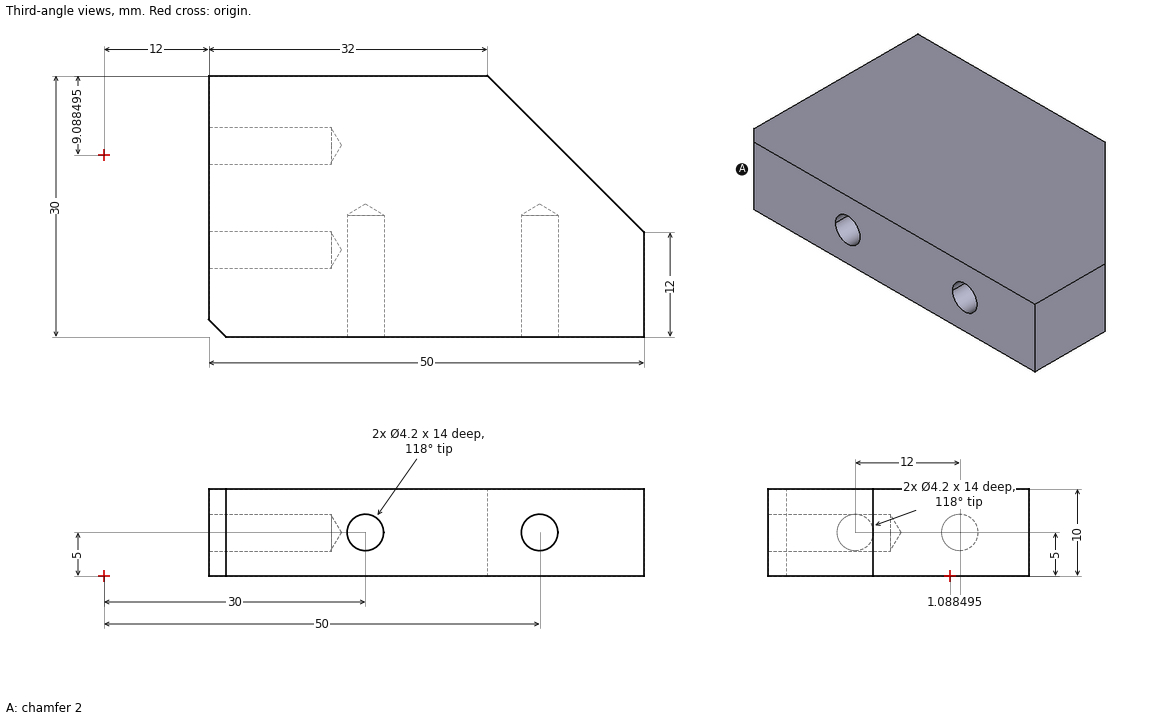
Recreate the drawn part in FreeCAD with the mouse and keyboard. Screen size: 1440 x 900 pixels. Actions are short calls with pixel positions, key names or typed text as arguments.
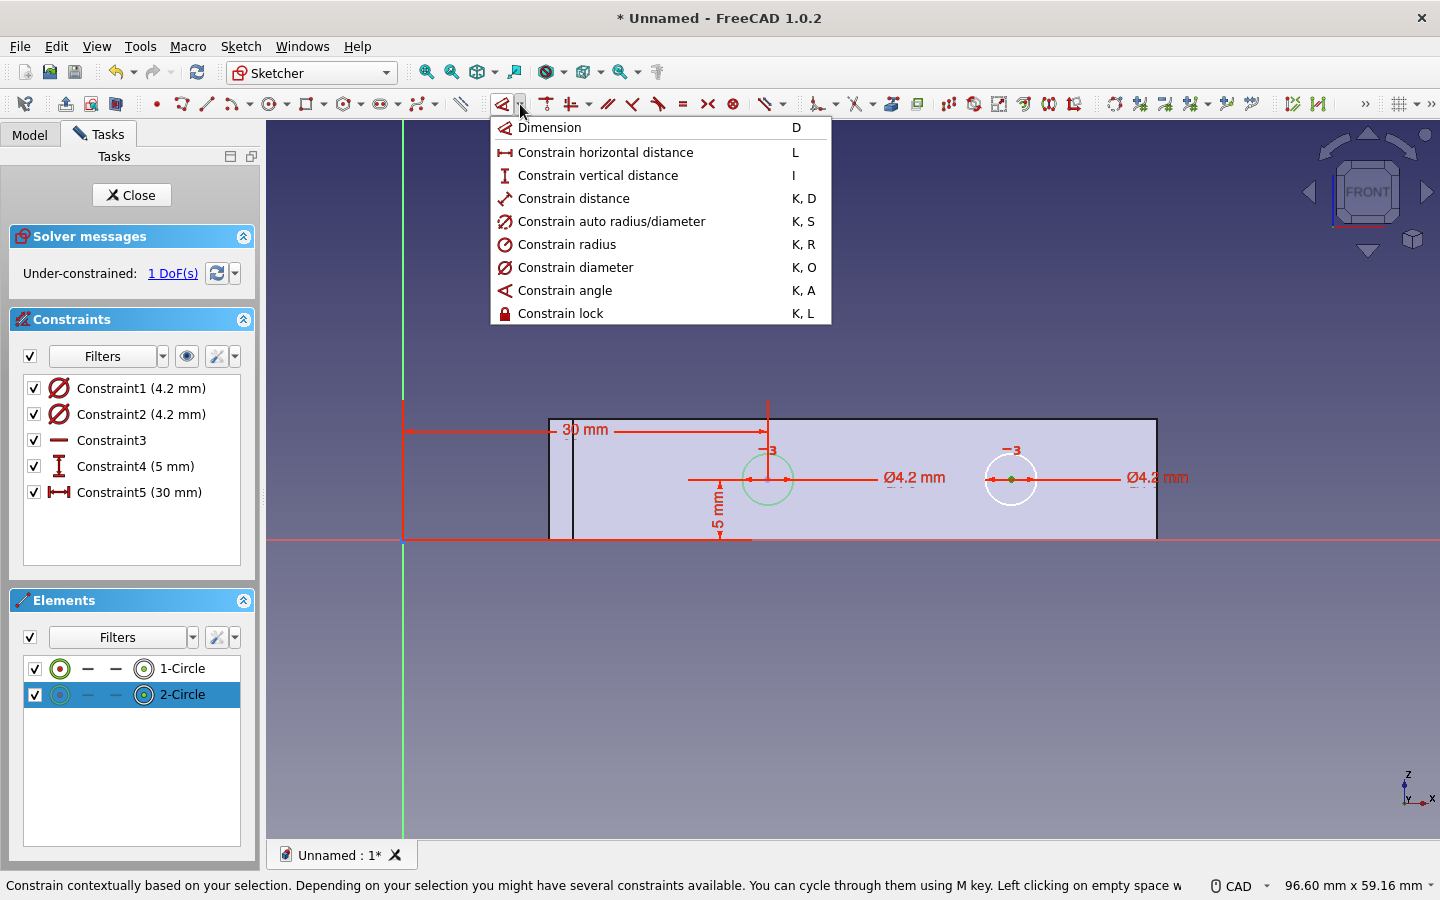
click(661, 152)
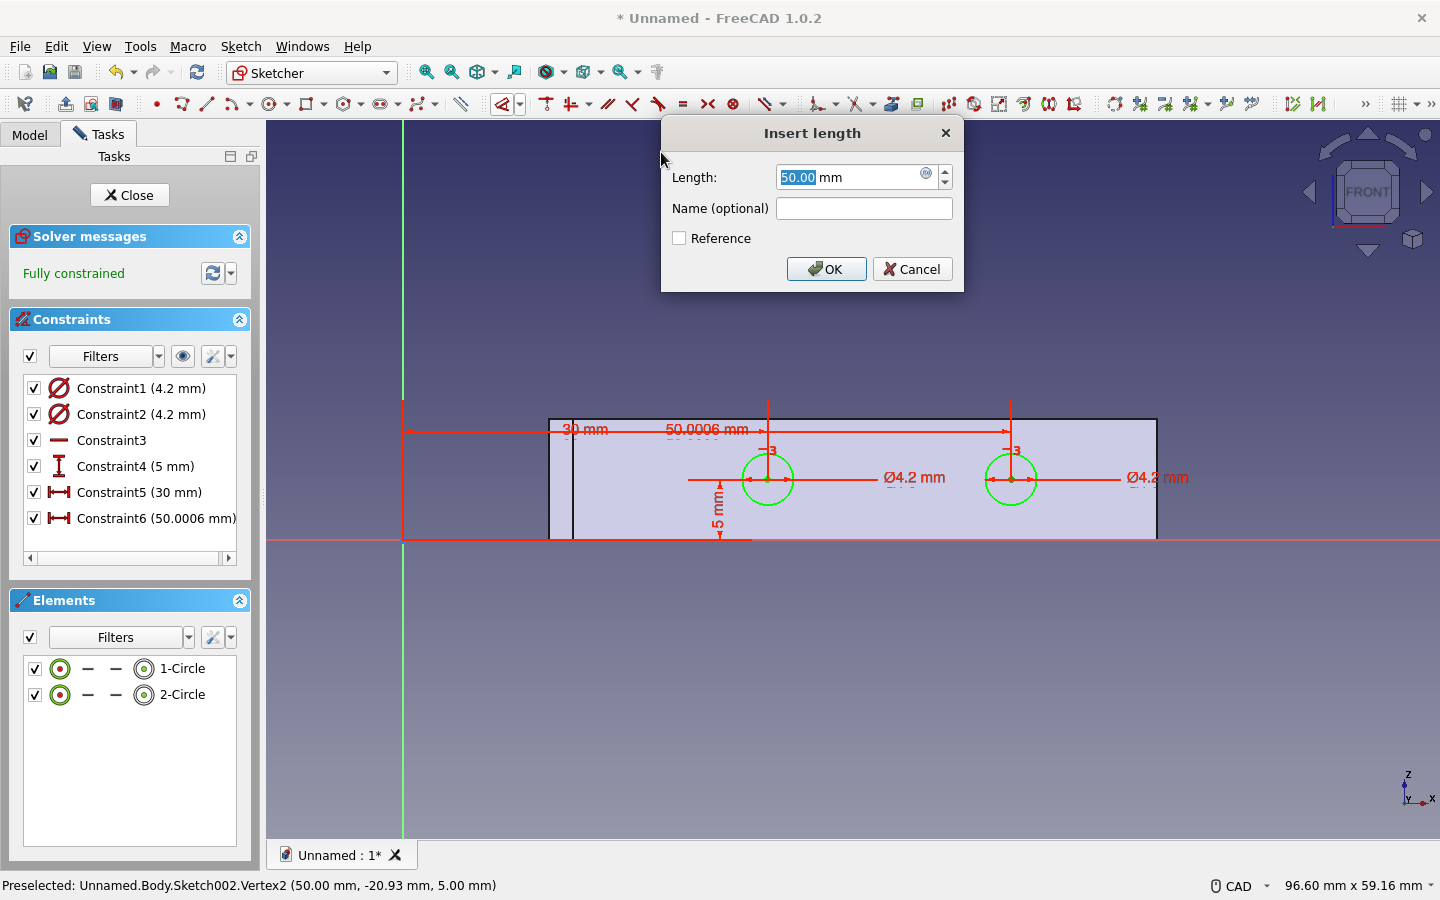
text(50)
key(Return)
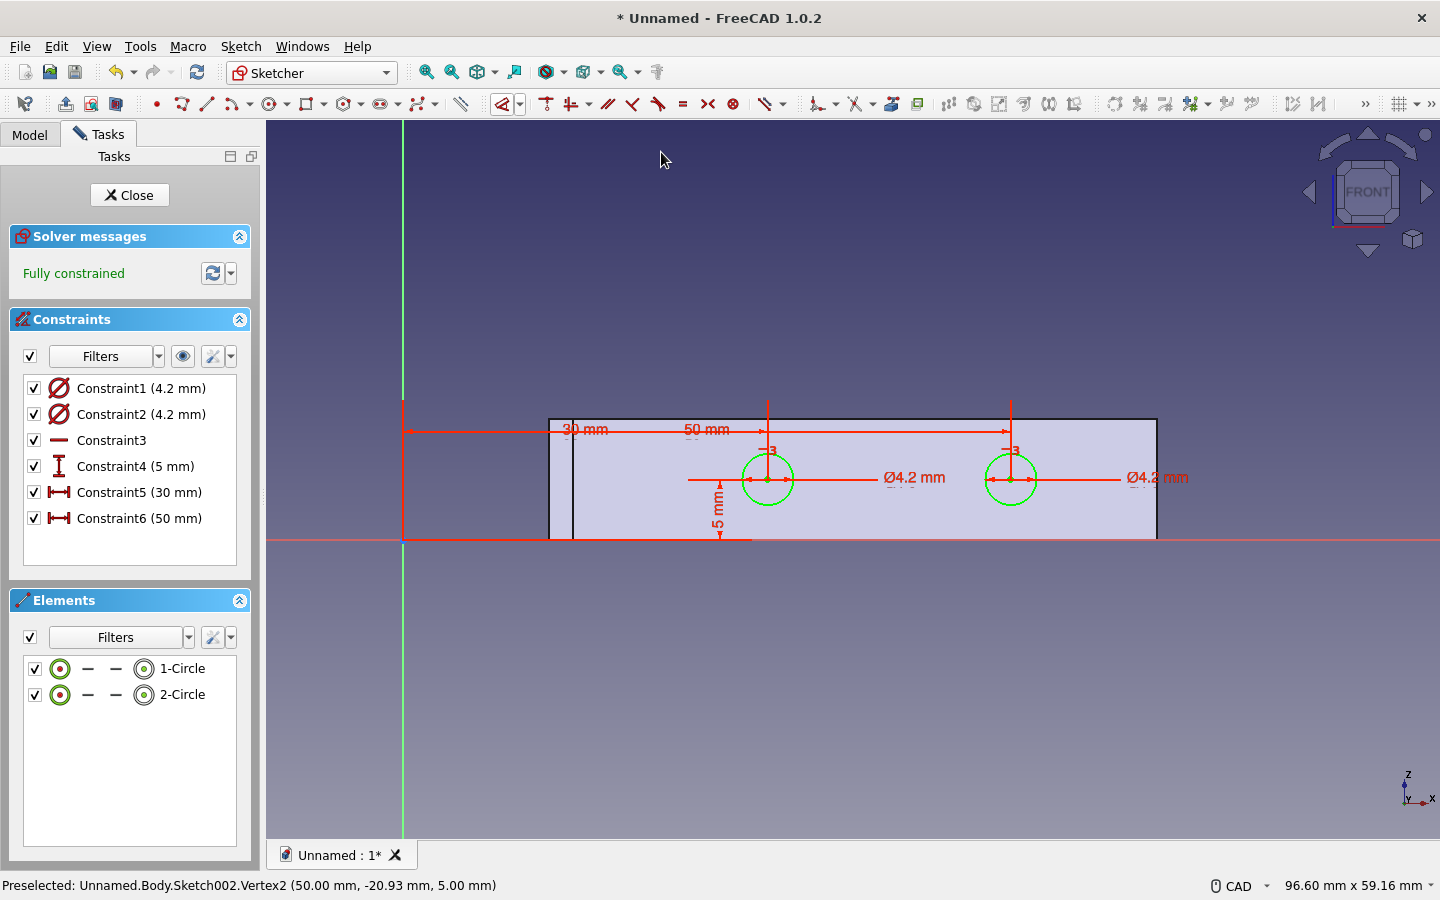
click(130, 195)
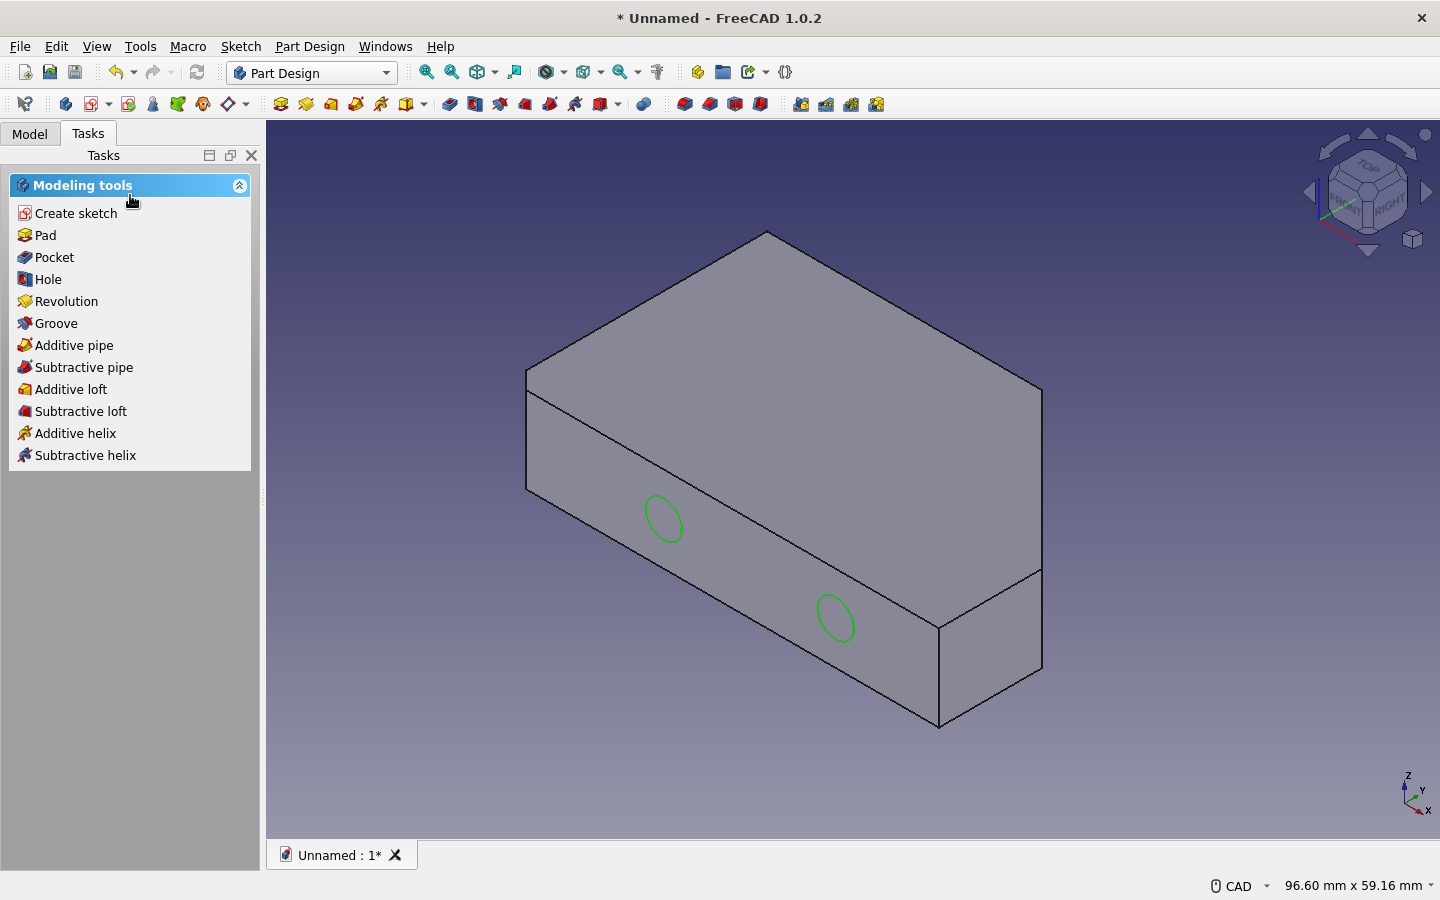
click(475, 104)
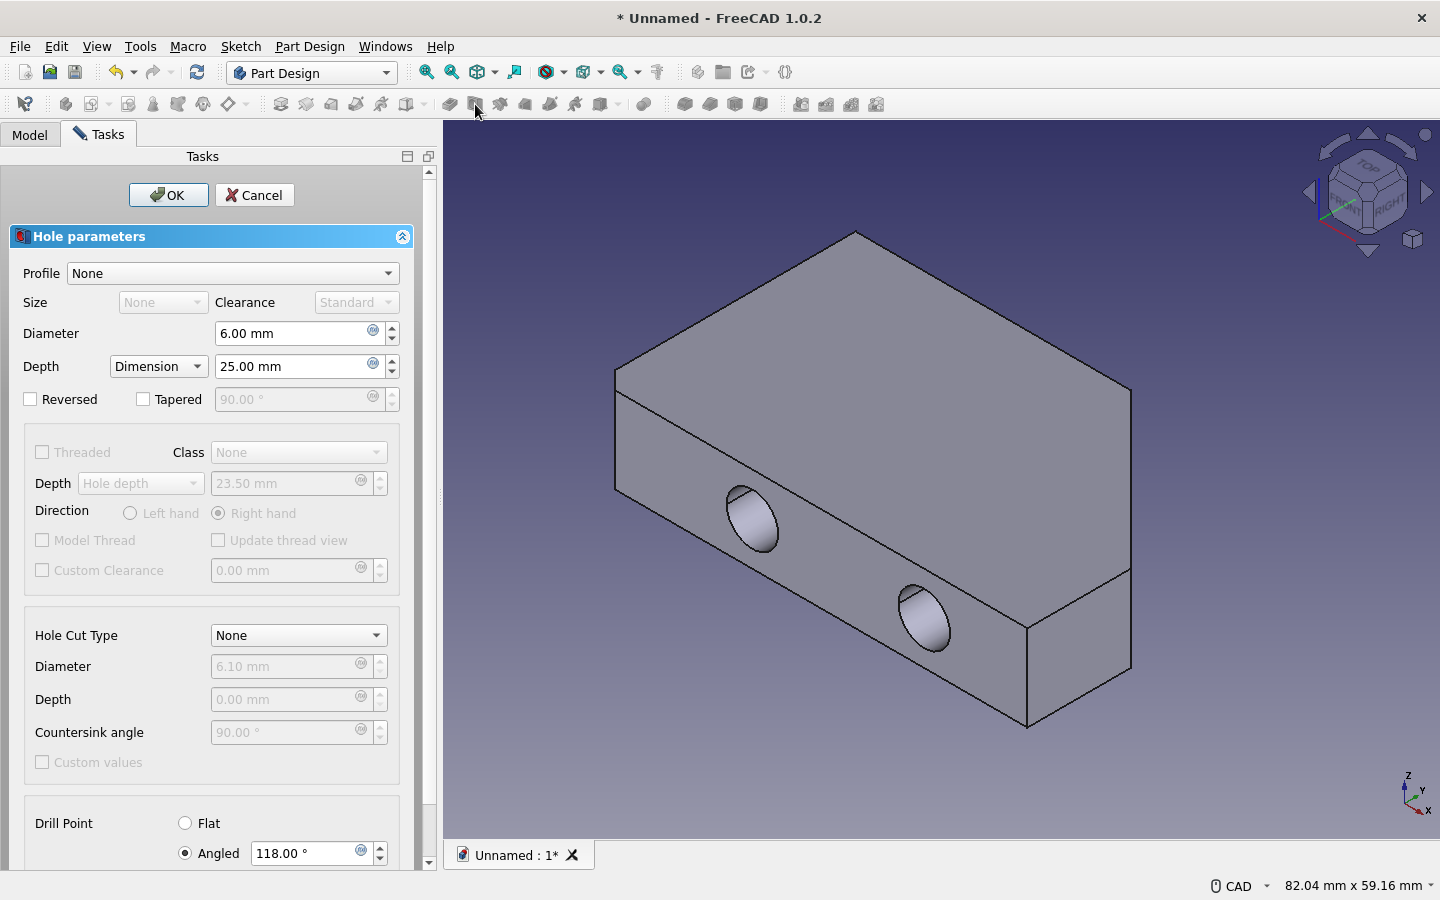
triple_click(300, 334)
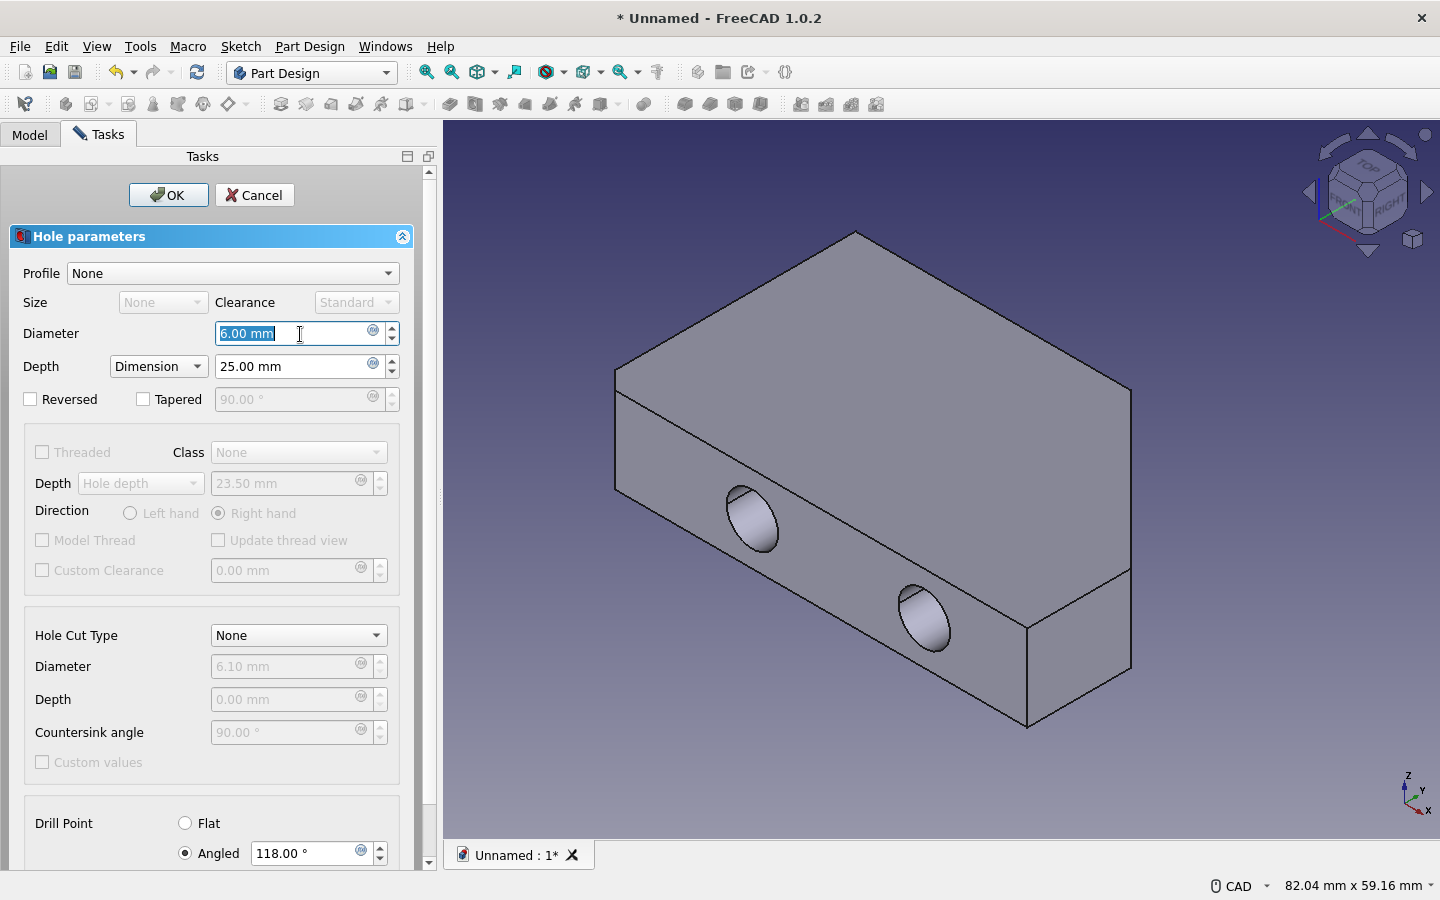
text(4.2)
key(Tab)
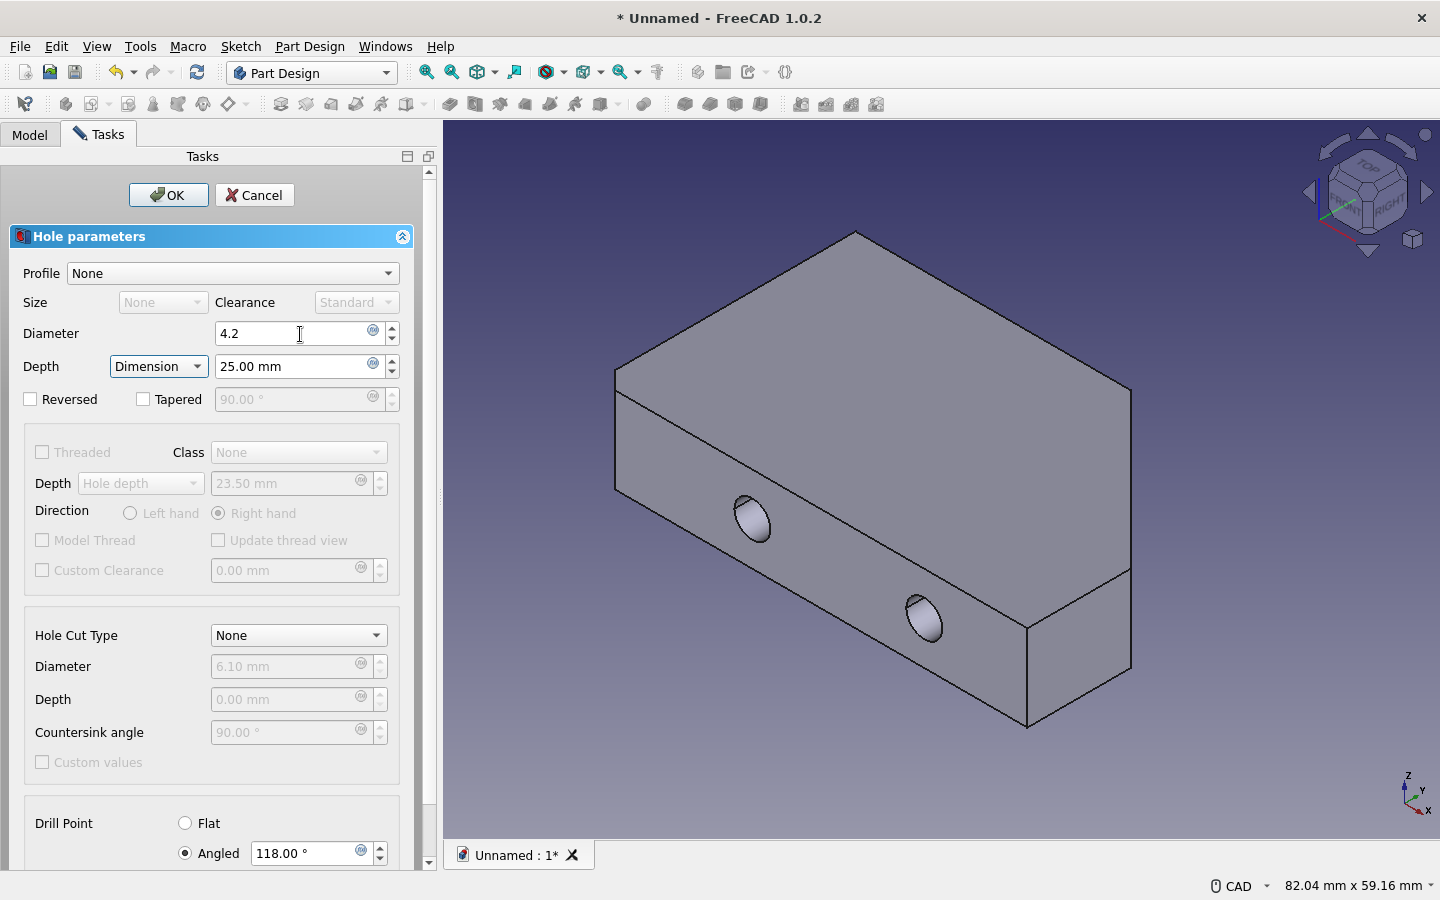
triple_click(300, 366)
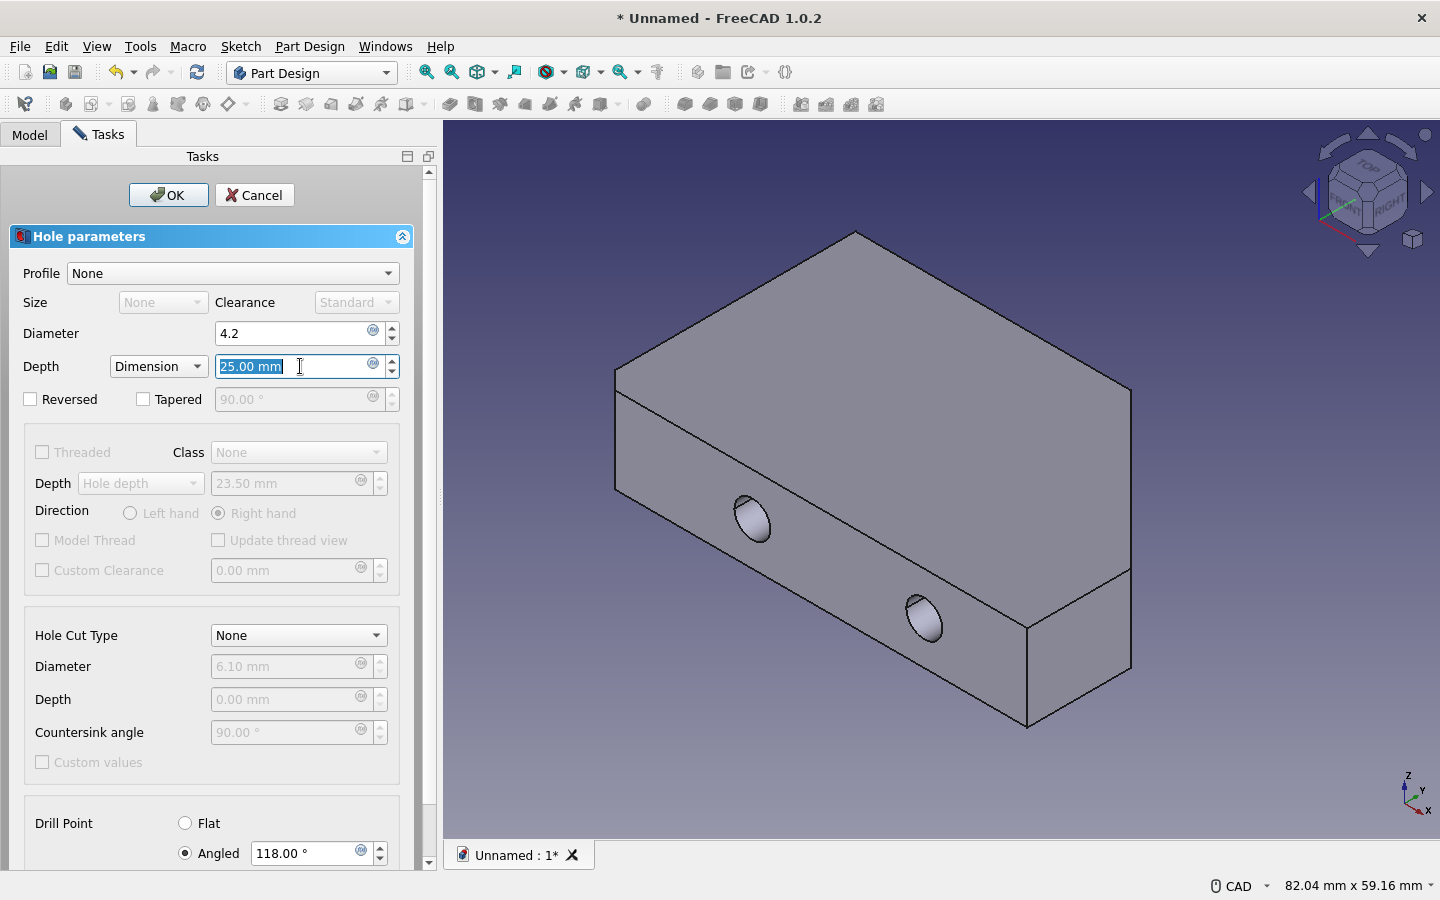
text(14)
key(Tab)